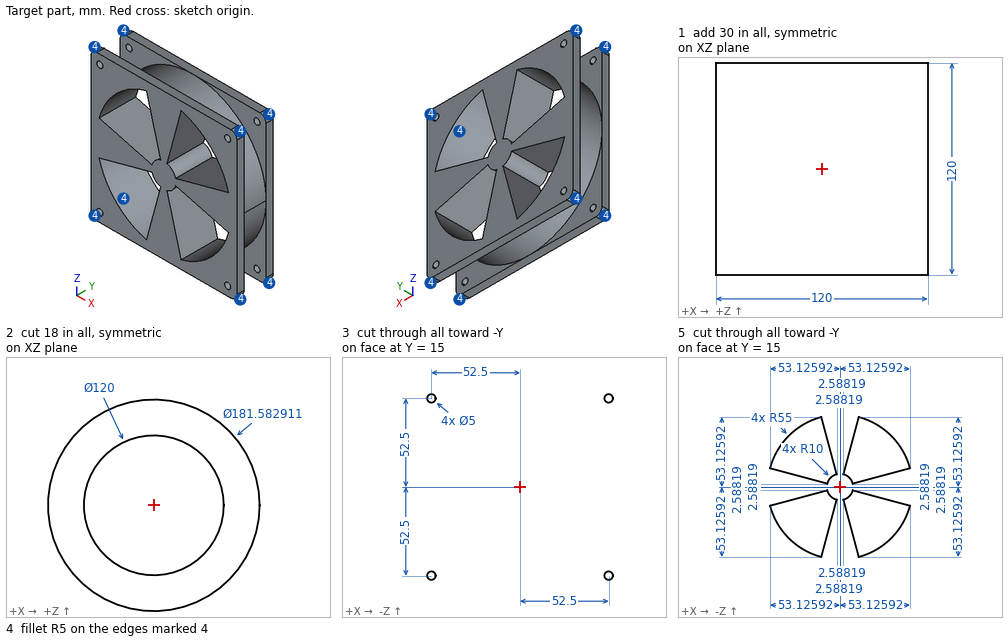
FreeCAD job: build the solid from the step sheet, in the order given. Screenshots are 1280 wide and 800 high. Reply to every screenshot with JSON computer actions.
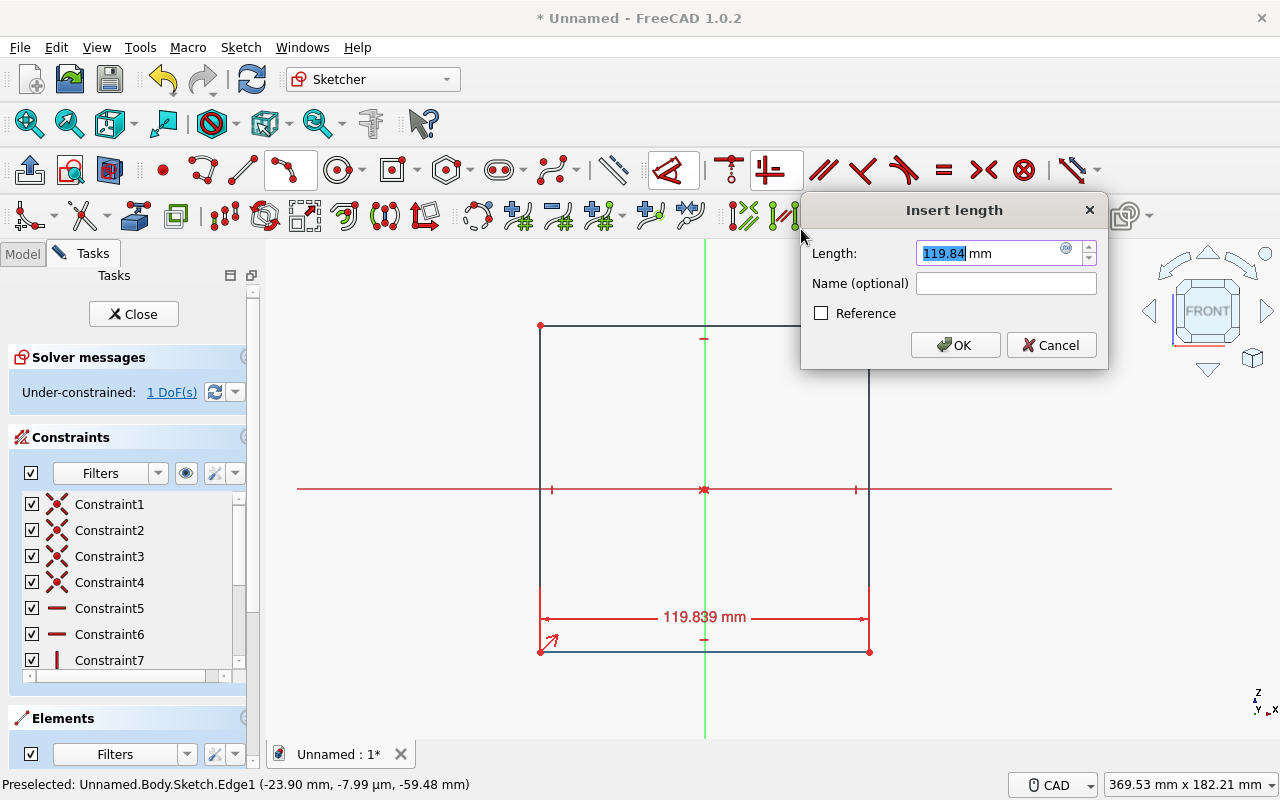
{"action": "type", "text": "120"}
{"action": "key", "text": "Return"}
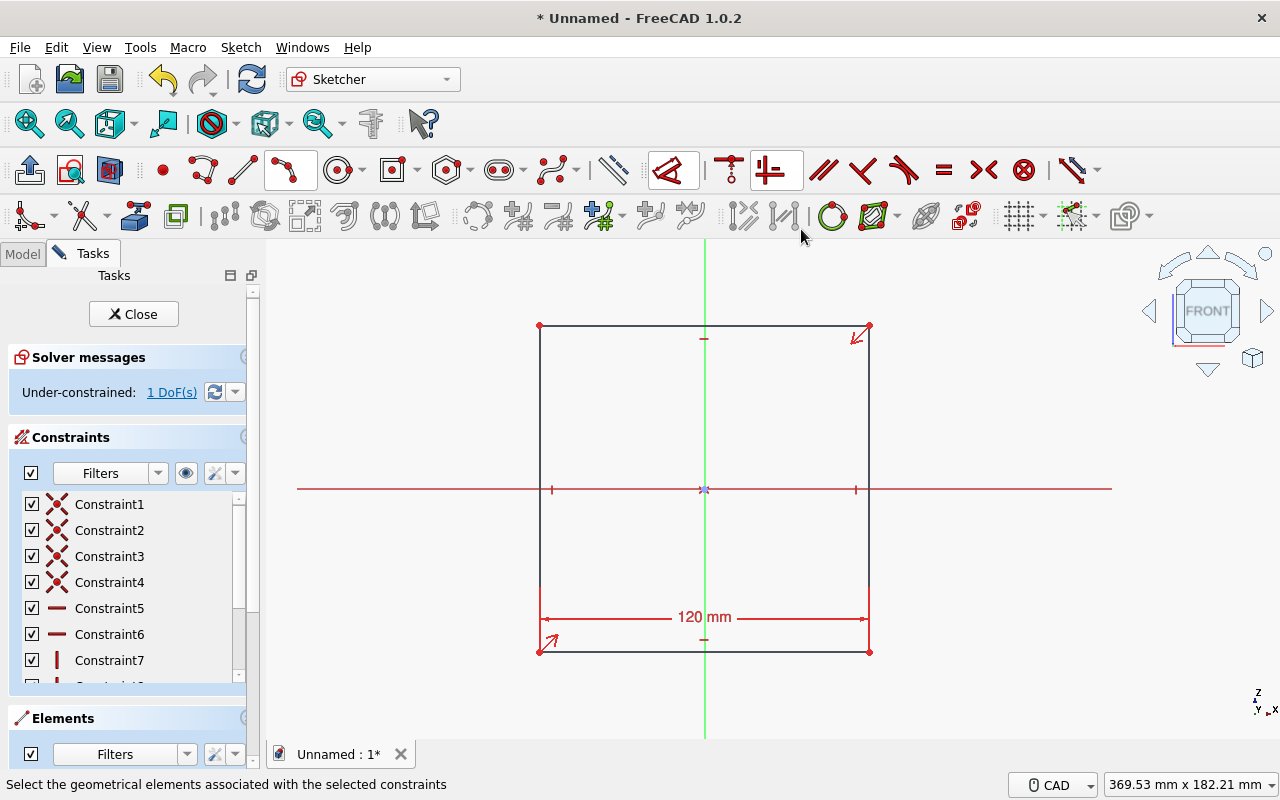
{"action": "left_click", "coordinate": [869, 555]}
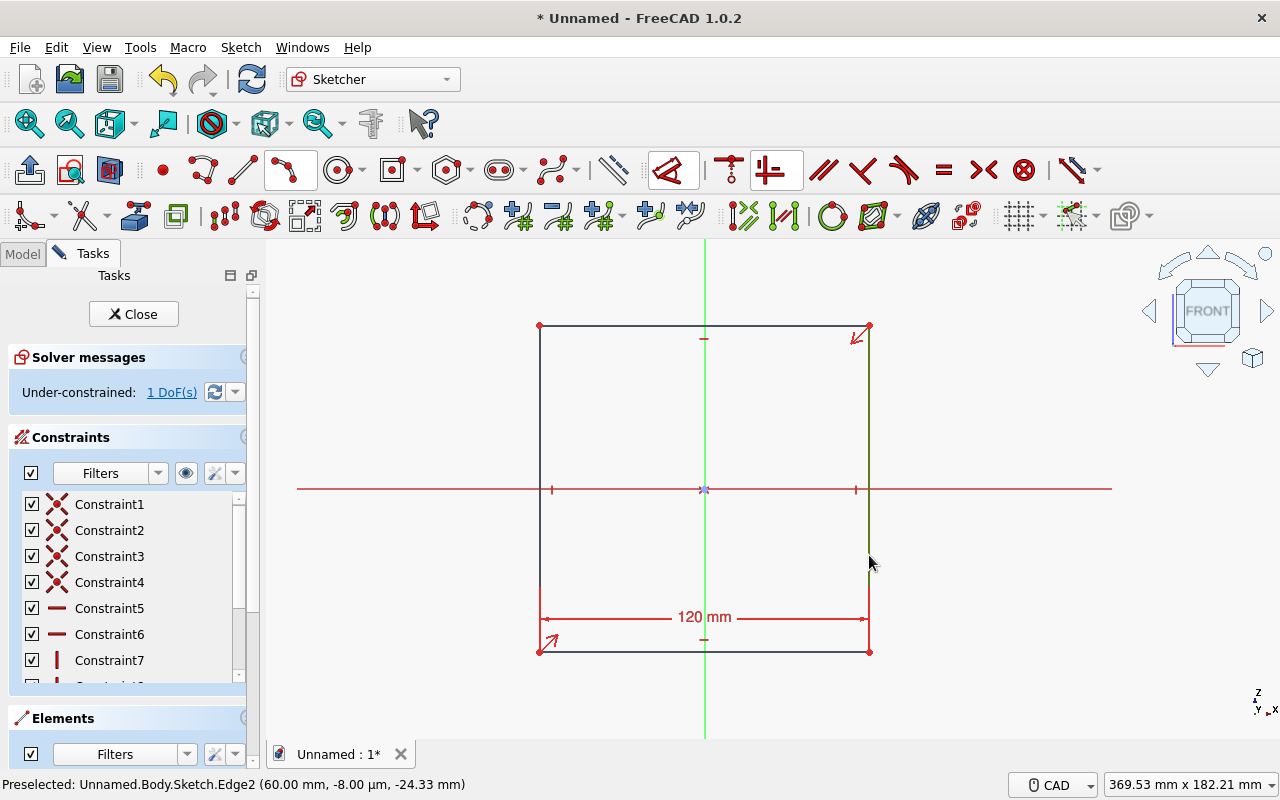
{"action": "left_click", "coordinate": [694, 170]}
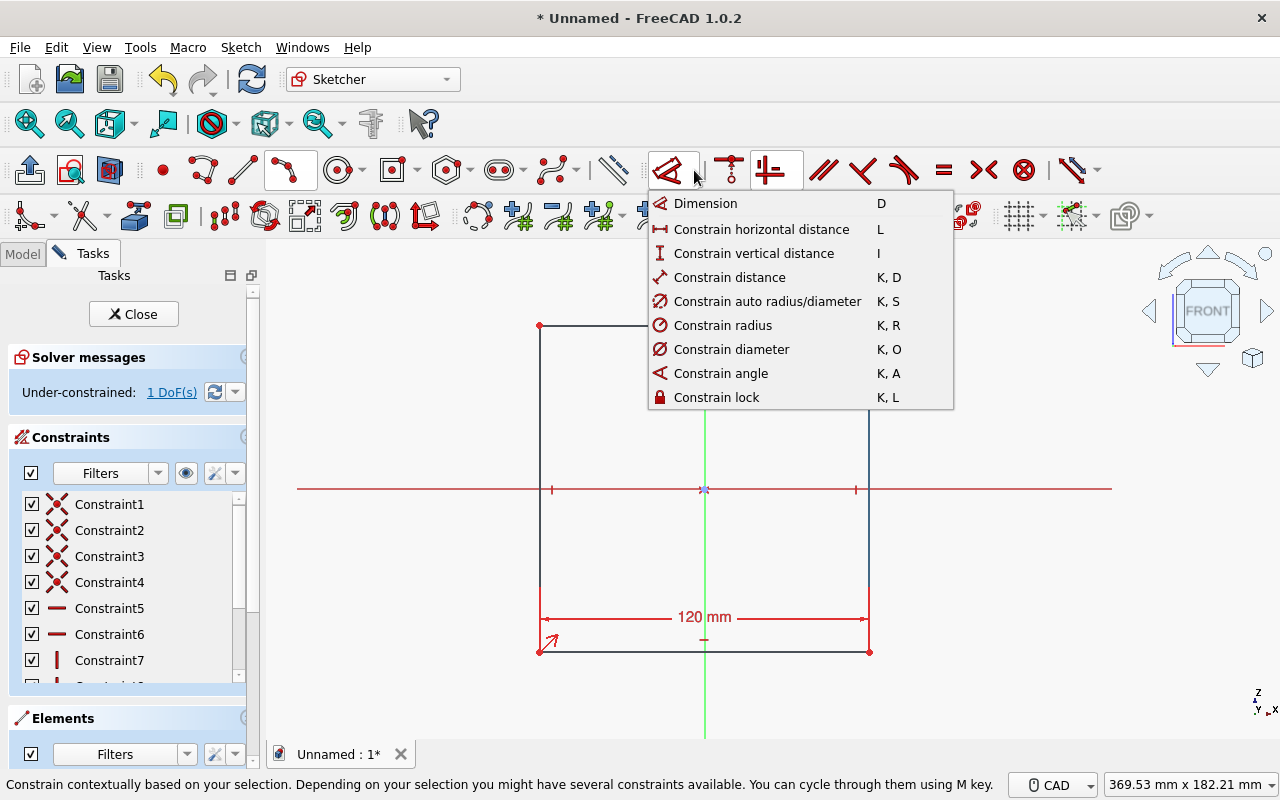
{"action": "left_click", "coordinate": [801, 253]}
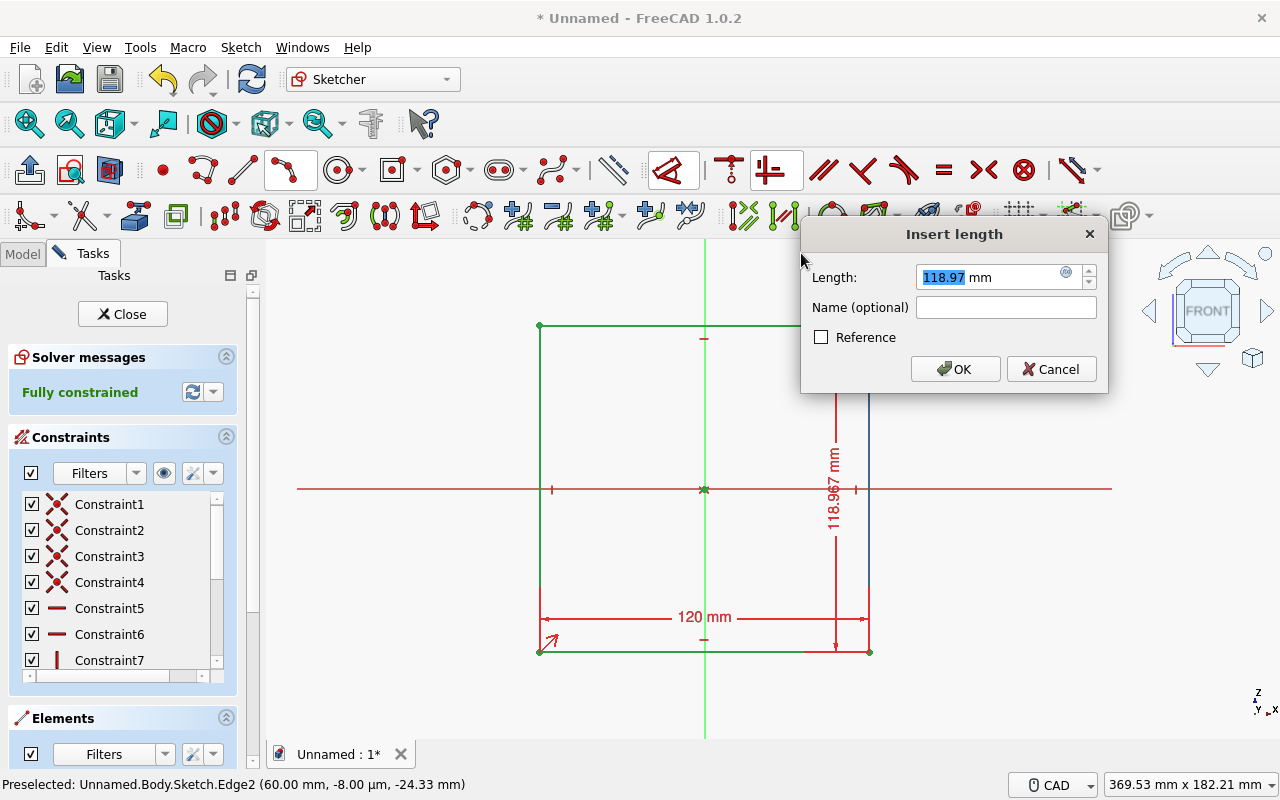
{"action": "type", "text": "120"}
{"action": "key", "text": "Return"}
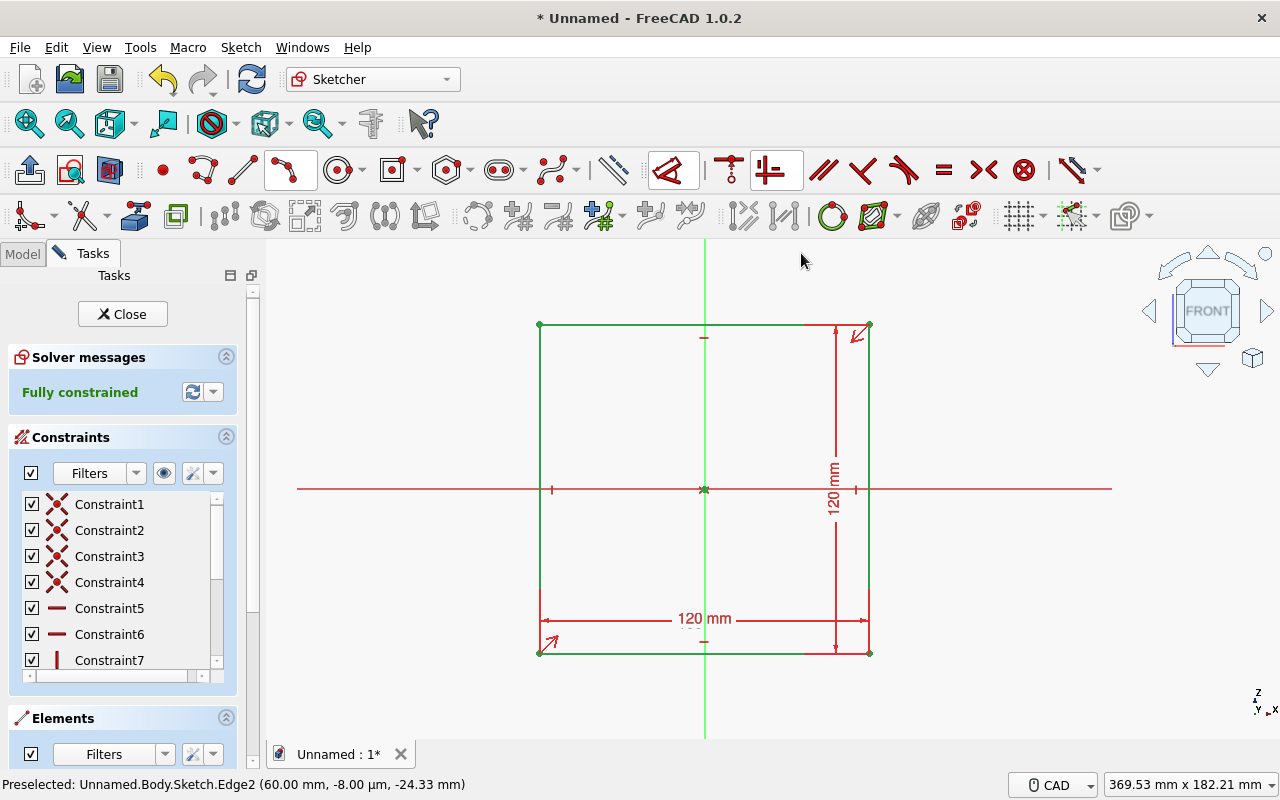
{"action": "left_click", "coordinate": [123, 314]}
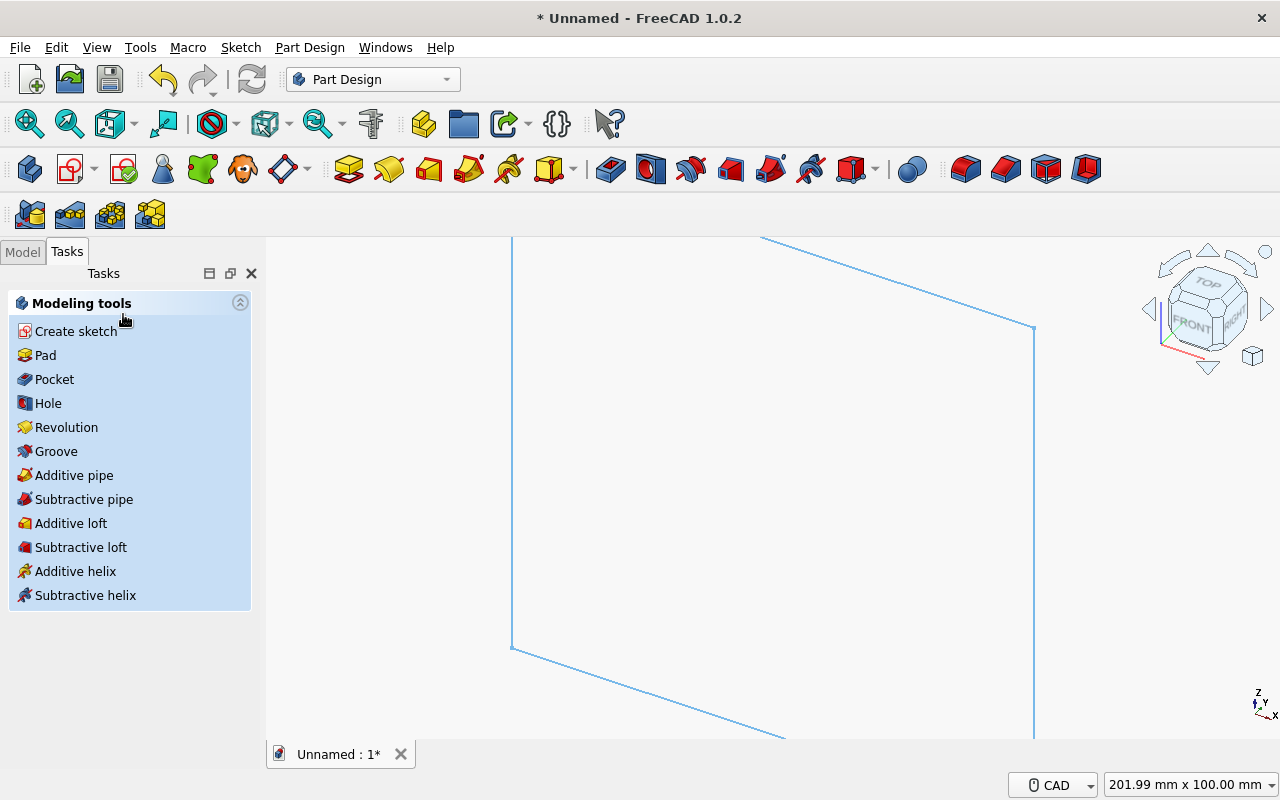
{"action": "left_click", "coordinate": [350, 170]}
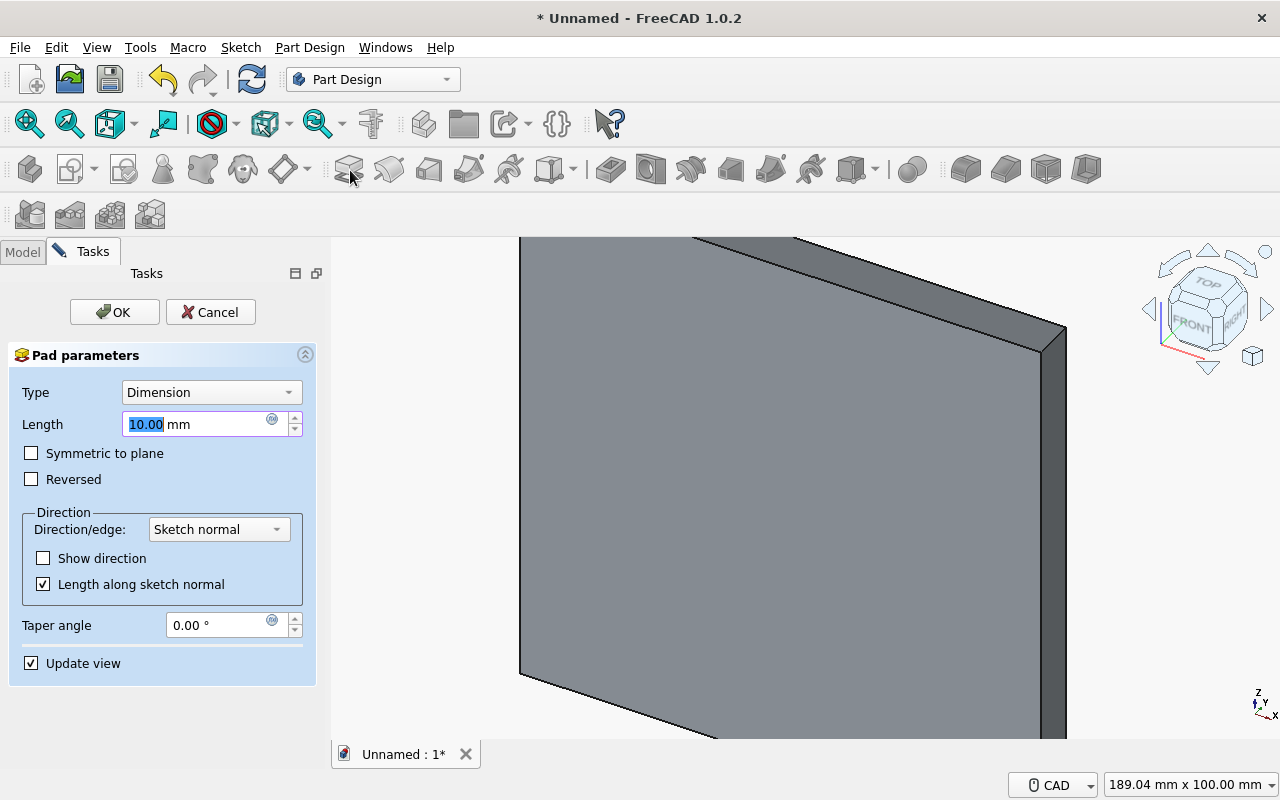
{"action": "type", "text": "30"}
{"action": "key", "text": "Tab"}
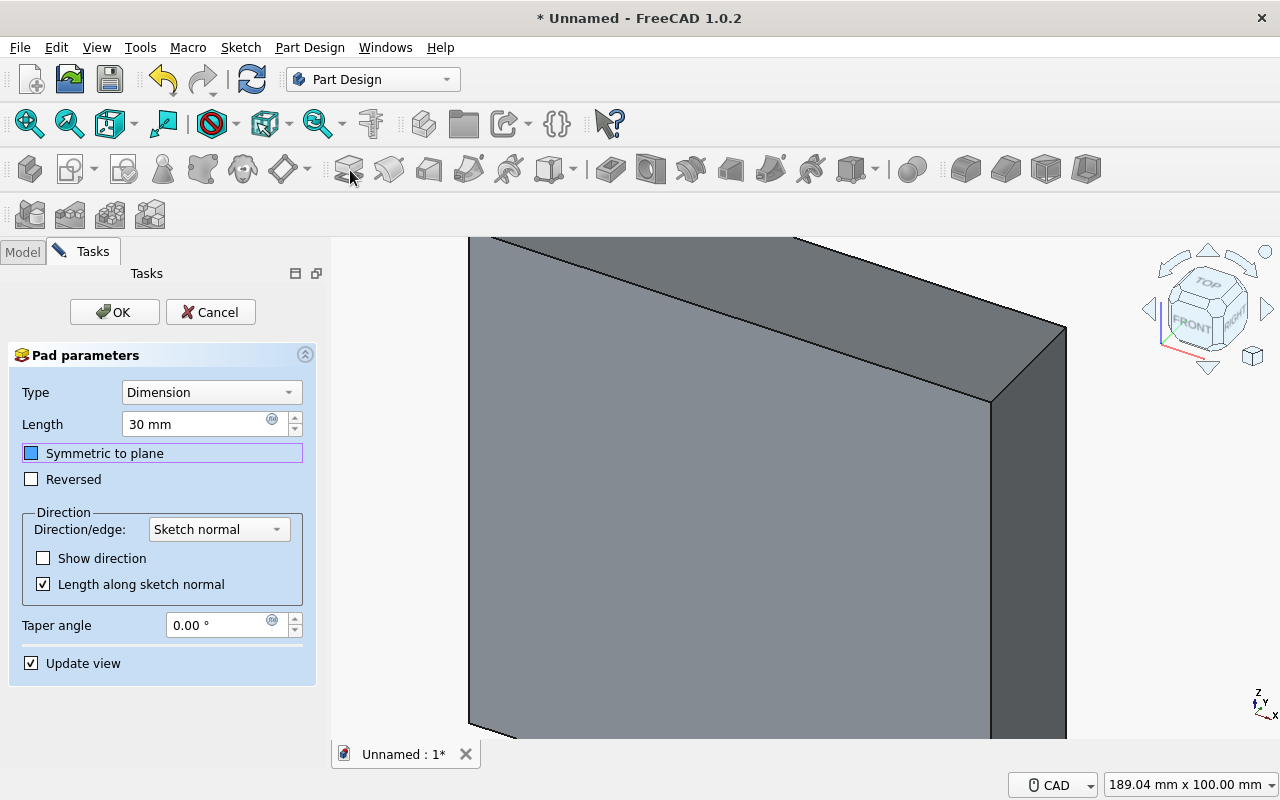
{"action": "left_click", "coordinate": [30, 453]}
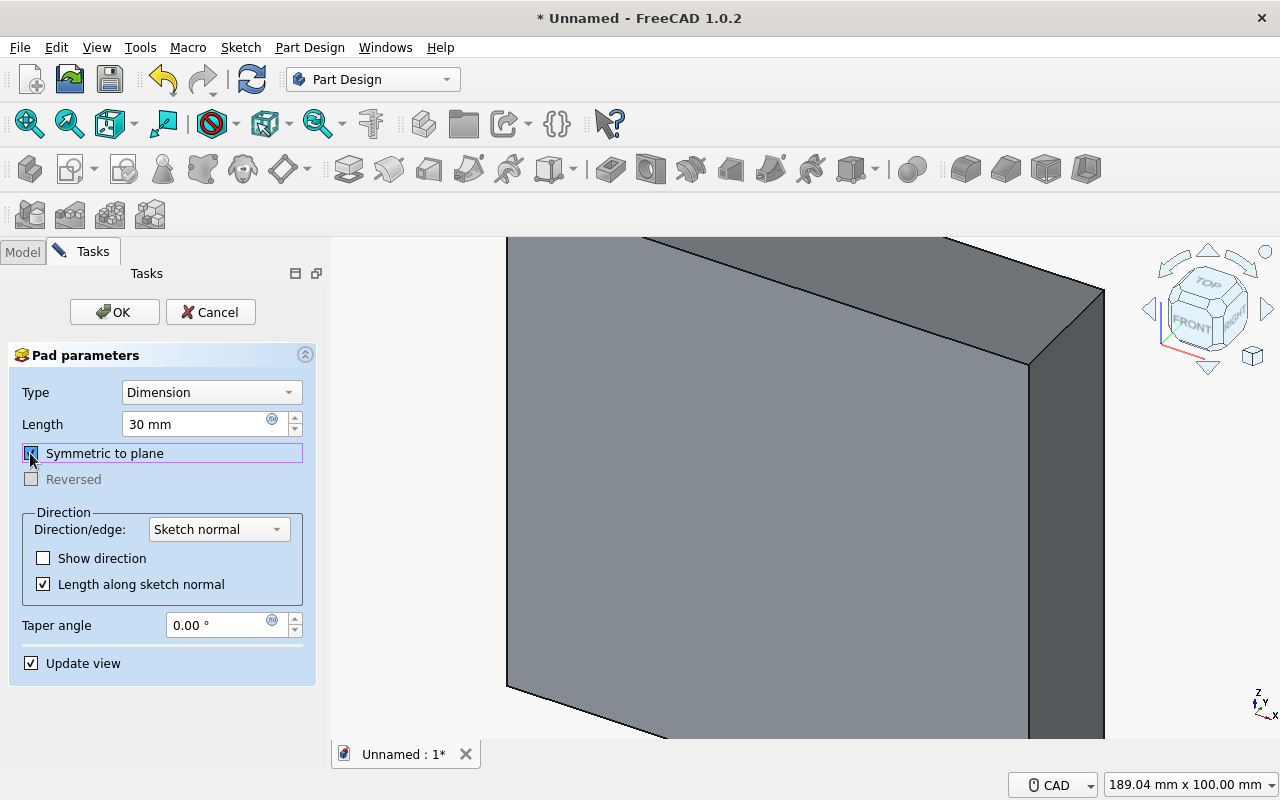
{"action": "left_click", "coordinate": [115, 312]}